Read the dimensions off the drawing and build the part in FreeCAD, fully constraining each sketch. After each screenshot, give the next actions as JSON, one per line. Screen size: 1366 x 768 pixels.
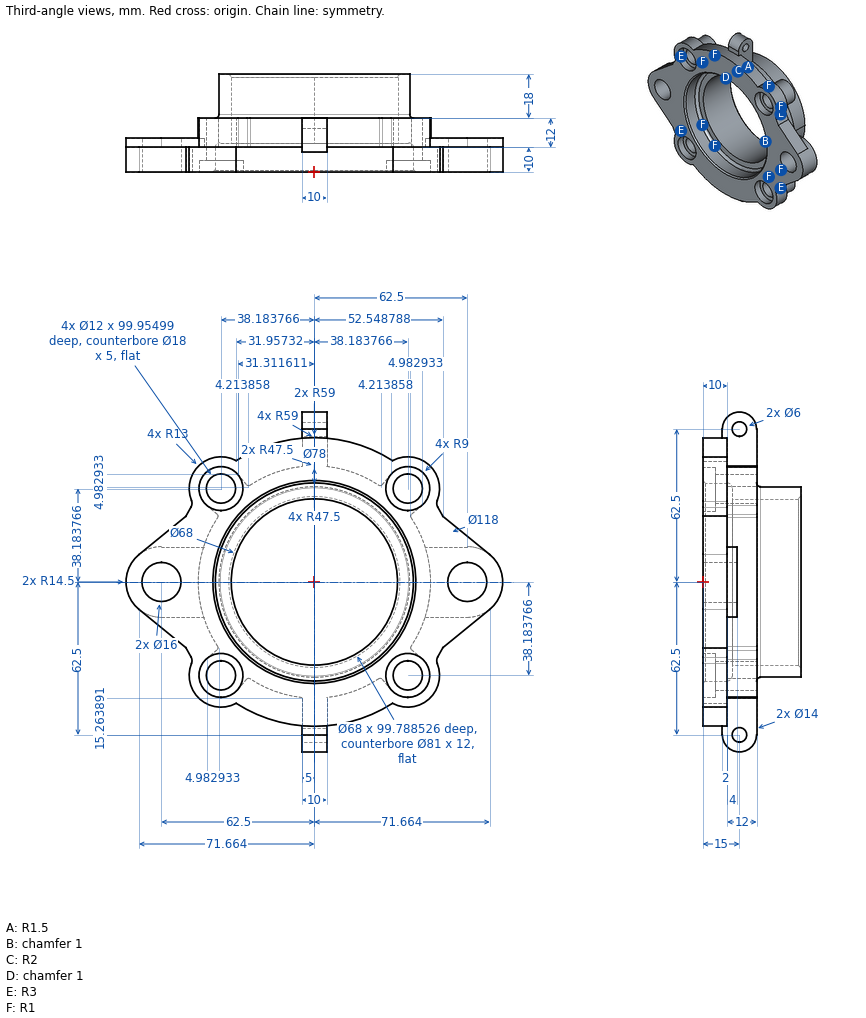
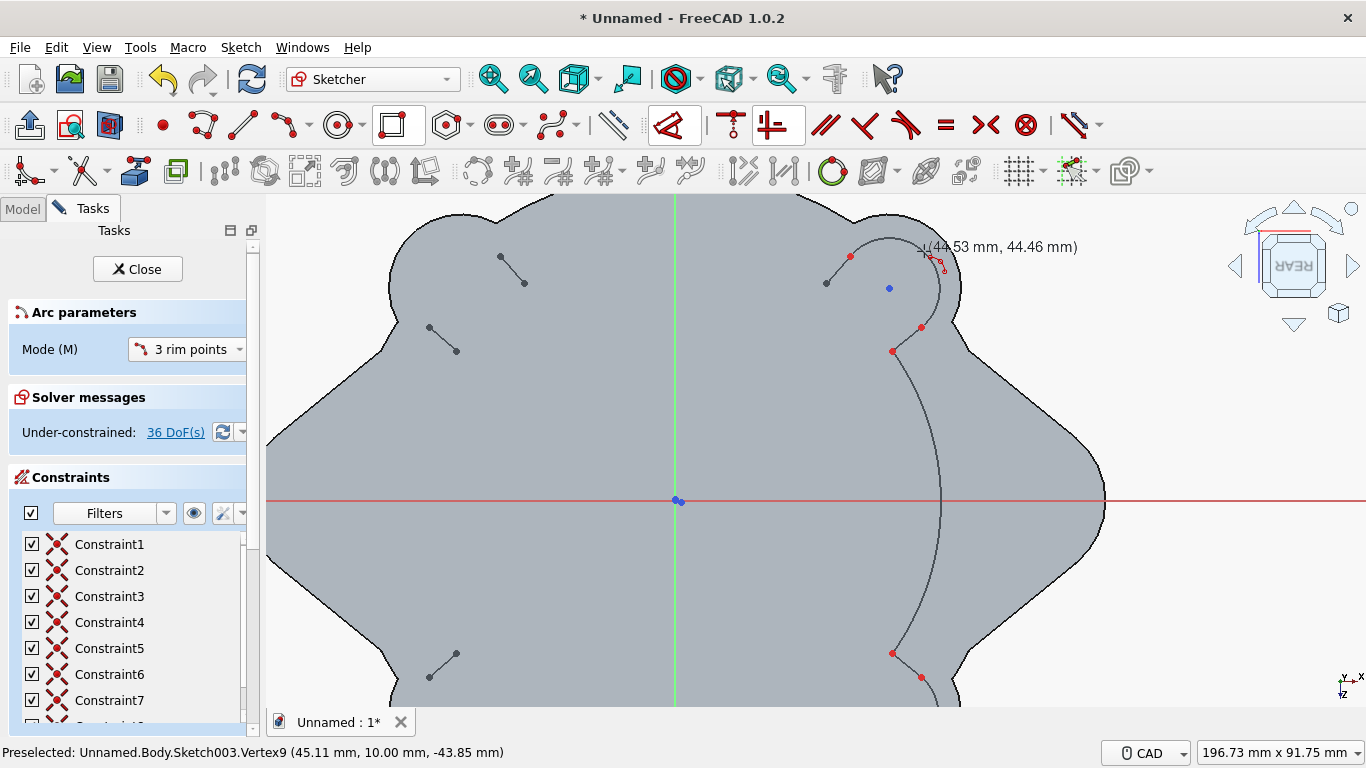
{"action": "left_click", "coordinate": [827, 284]}
{"action": "left_click", "coordinate": [524, 284]}
{"action": "left_click", "coordinate": [707, 237]}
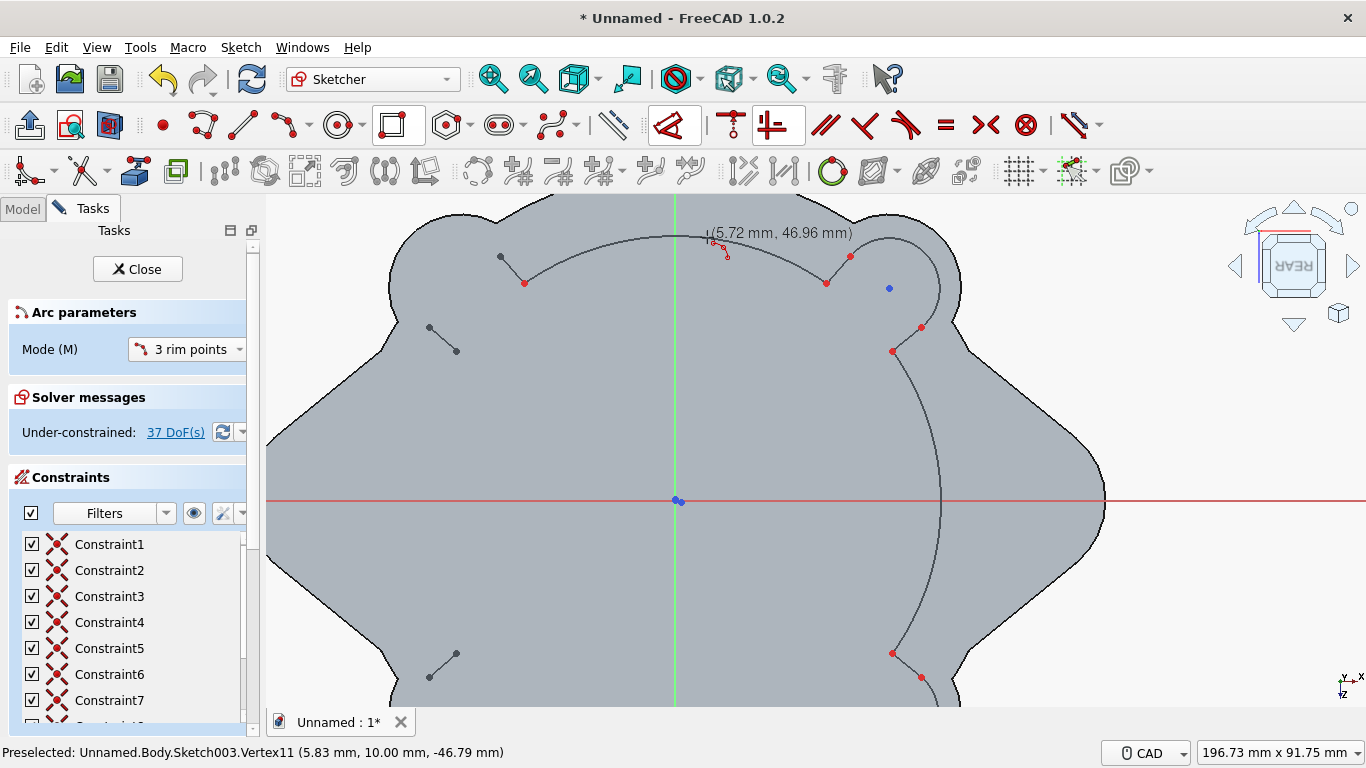
{"action": "left_click", "coordinate": [501, 256]}
{"action": "left_click", "coordinate": [430, 327]}
{"action": "left_click", "coordinate": [426, 251]}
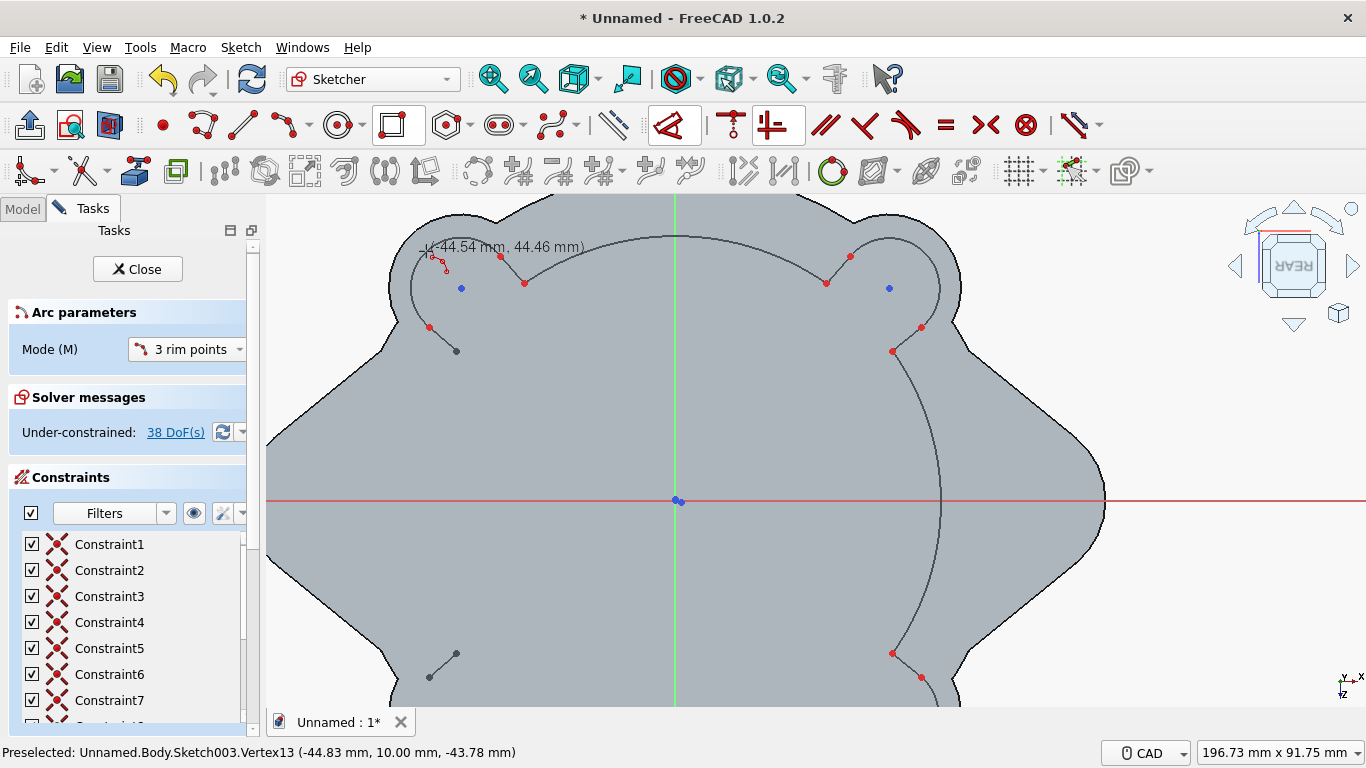
{"action": "left_click", "coordinate": [457, 351]}
{"action": "left_click", "coordinate": [457, 654]}
{"action": "left_click", "coordinate": [411, 468]}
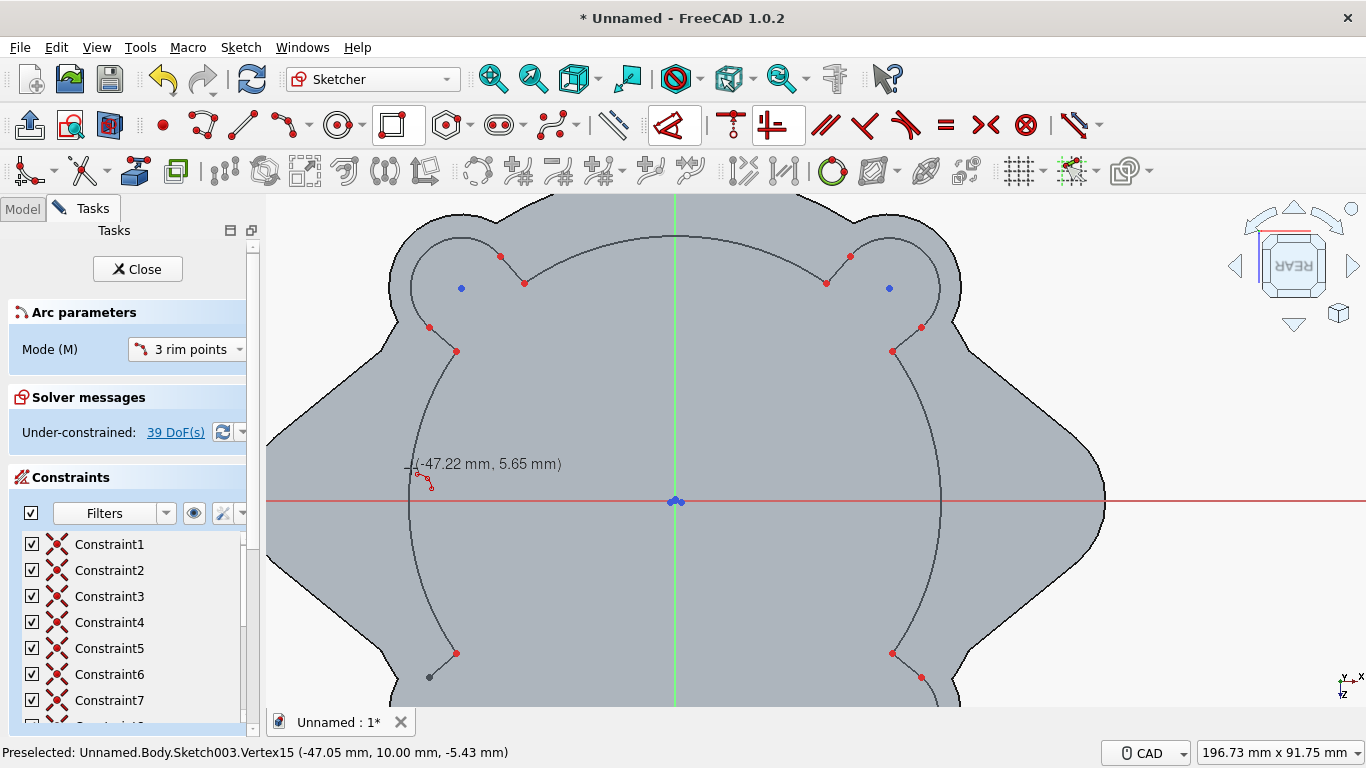
{"action": "left_click", "coordinate": [430, 677]}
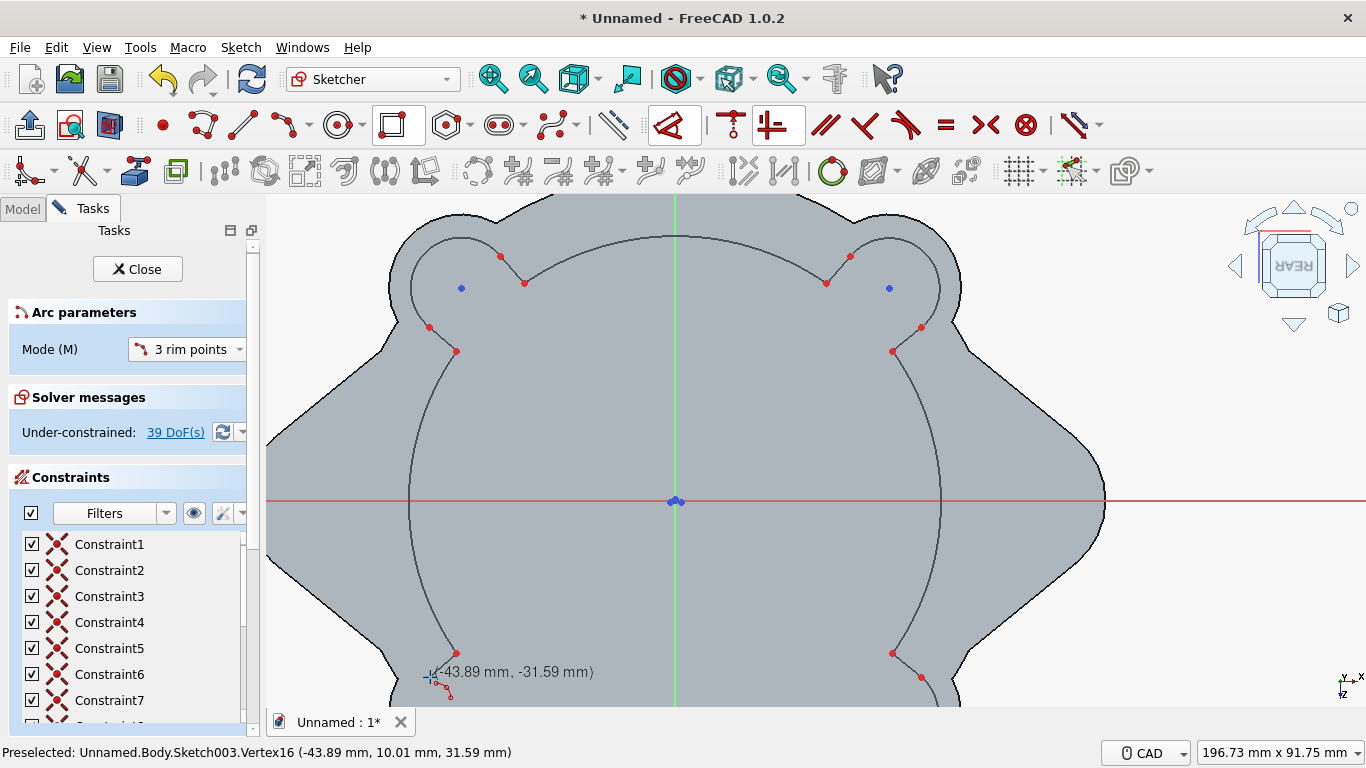
{"action": "scroll", "coordinate": [895, 349], "scroll_direction": "down", "scroll_amount": 2}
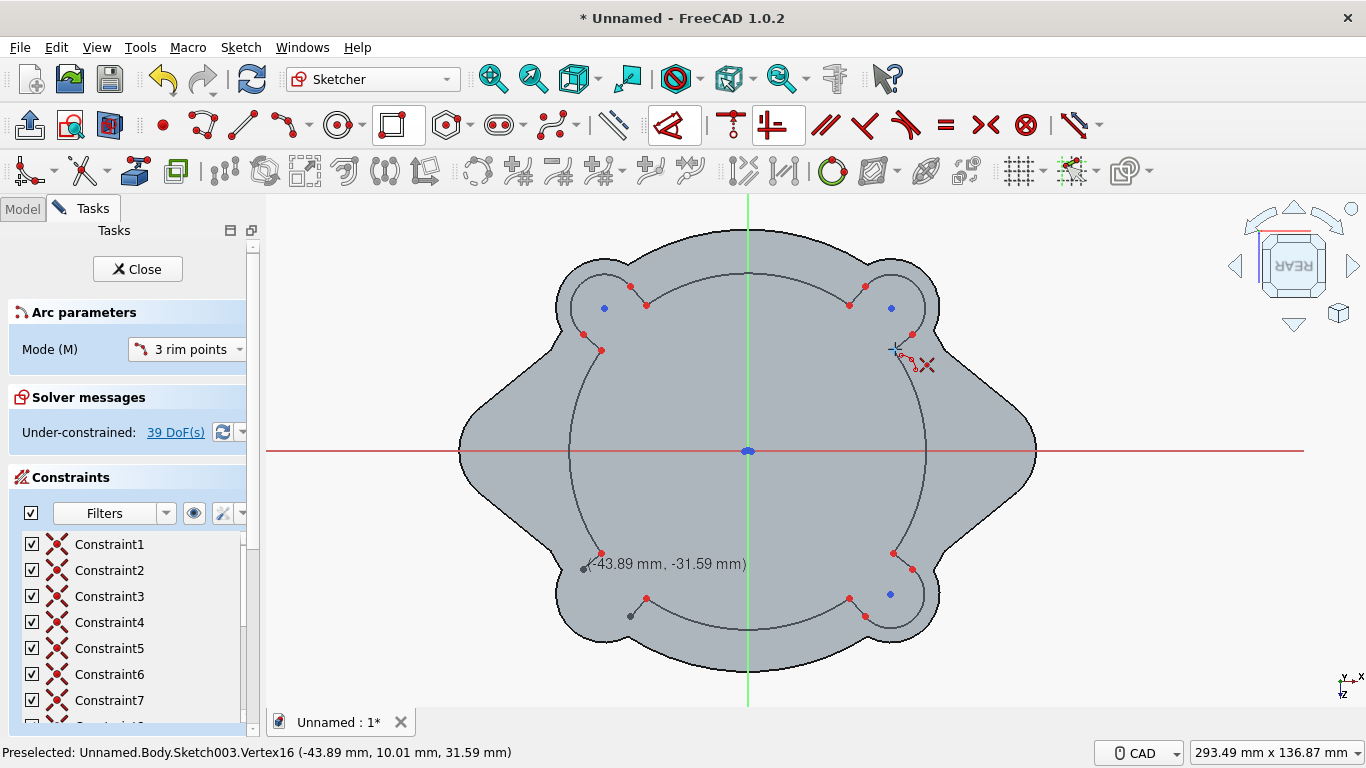
{"action": "scroll", "coordinate": [630, 616], "scroll_direction": "up", "scroll_amount": 2}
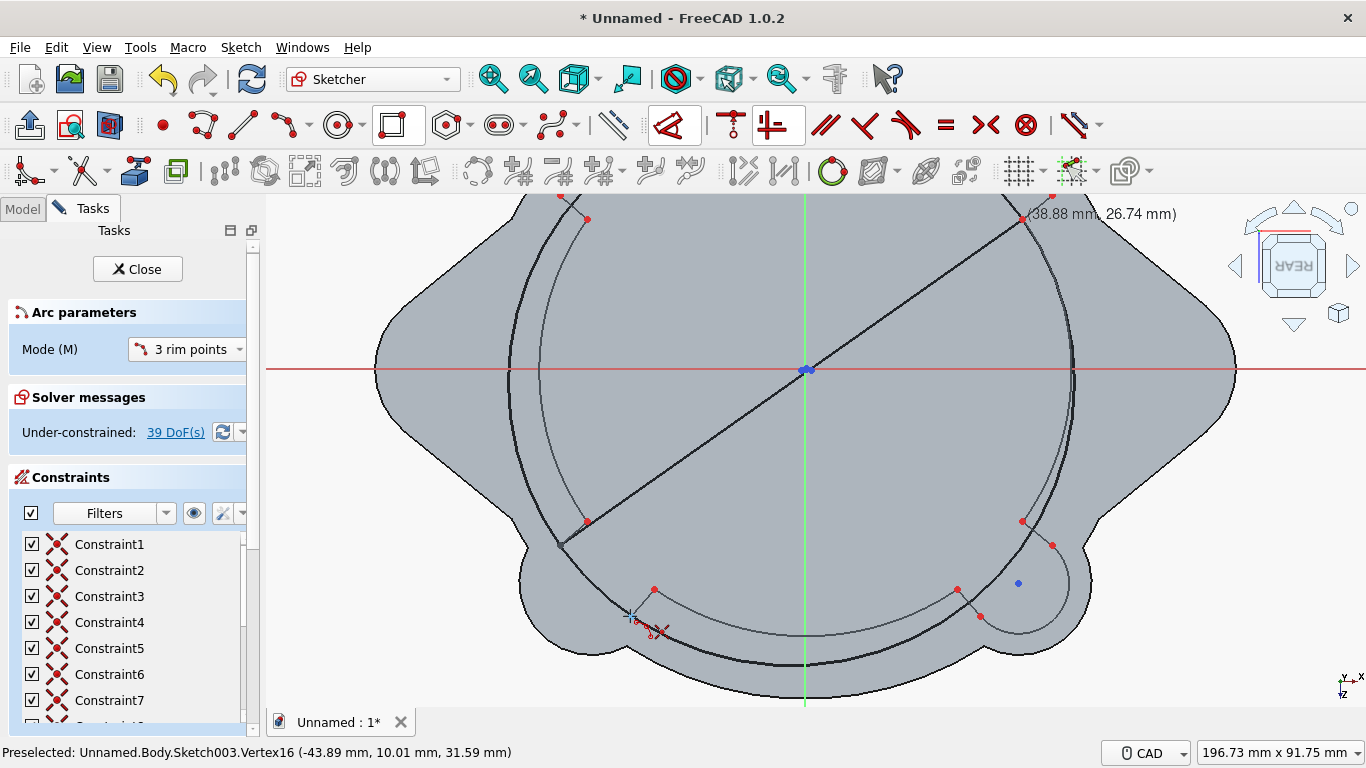
{"action": "left_click", "coordinate": [631, 617]}
{"action": "left_click", "coordinate": [556, 618]}
{"action": "key", "text": "Escape"}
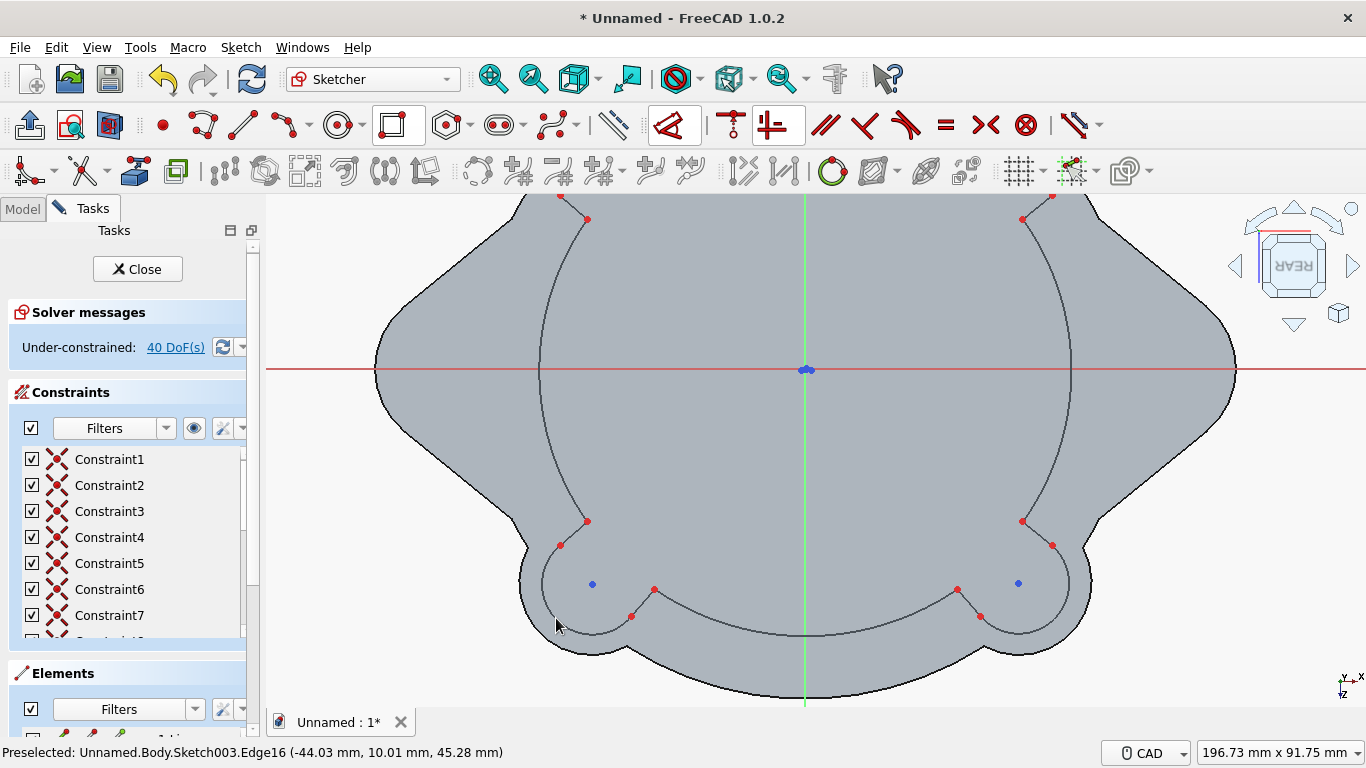
{"action": "scroll", "coordinate": [638, 608], "scroll_direction": "up", "scroll_amount": 2}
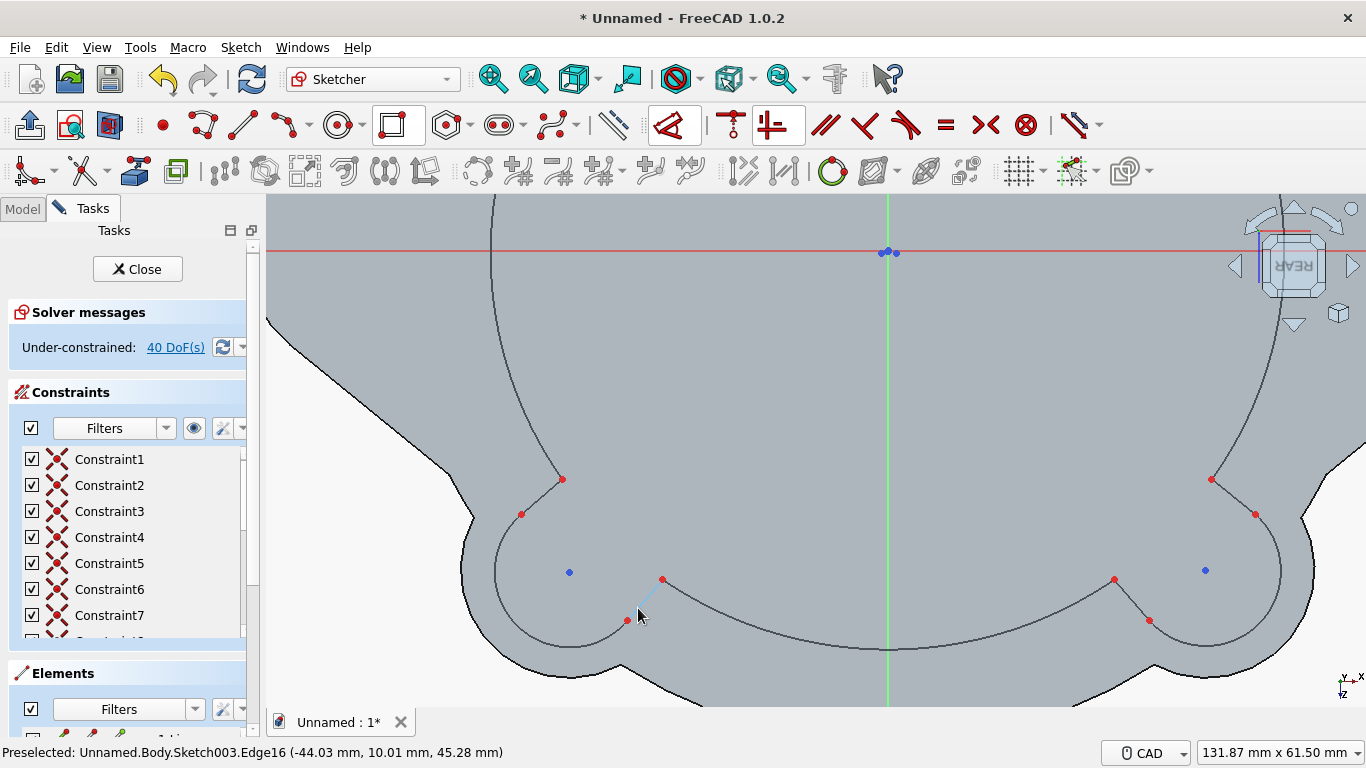
{"action": "left_click", "coordinate": [638, 608]}